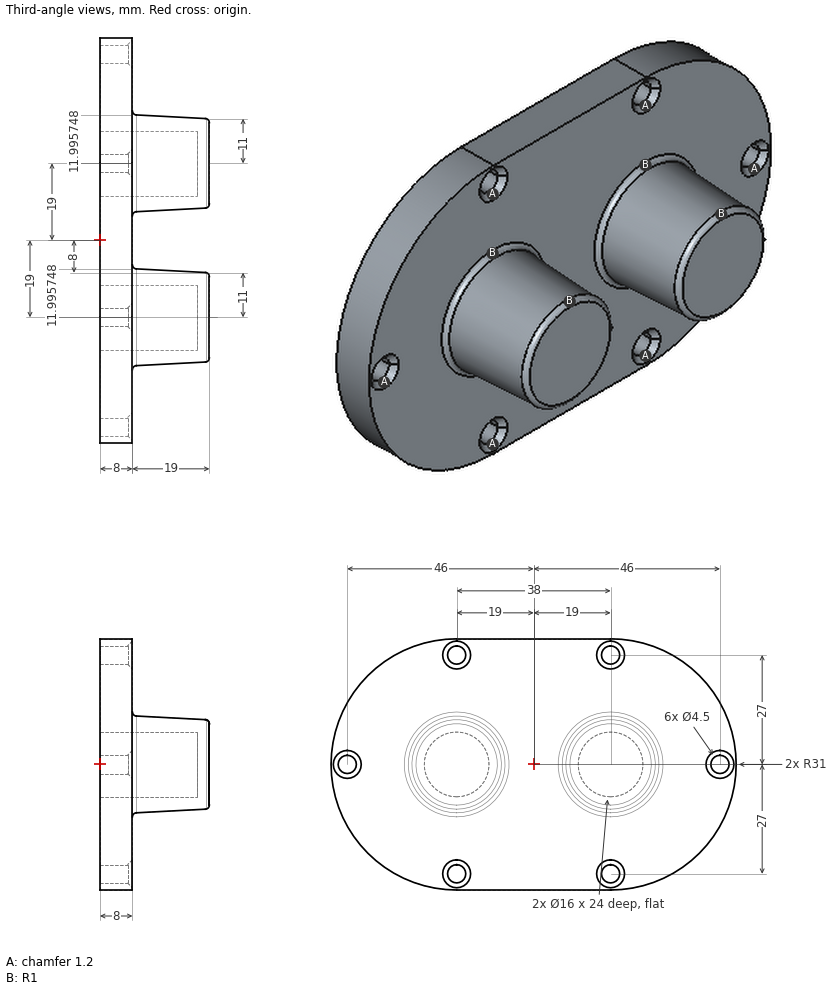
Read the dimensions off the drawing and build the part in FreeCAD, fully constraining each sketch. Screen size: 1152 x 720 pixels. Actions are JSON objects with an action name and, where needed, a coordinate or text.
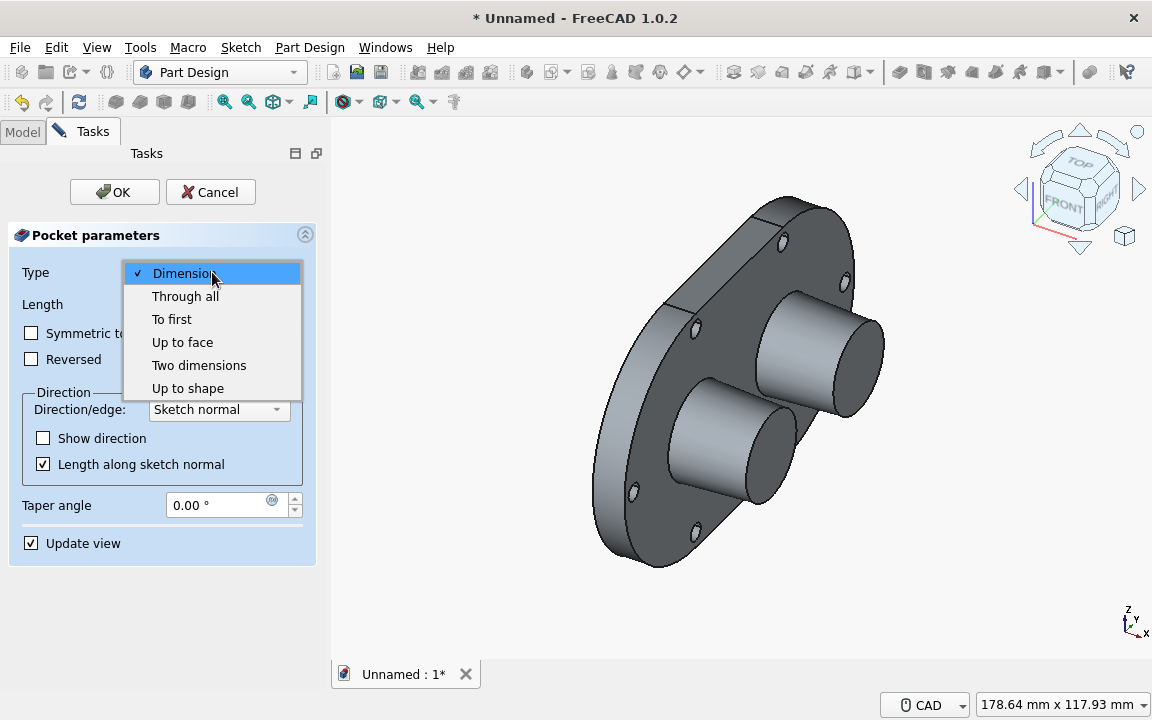
{"action": "left_click", "coordinate": [212, 296]}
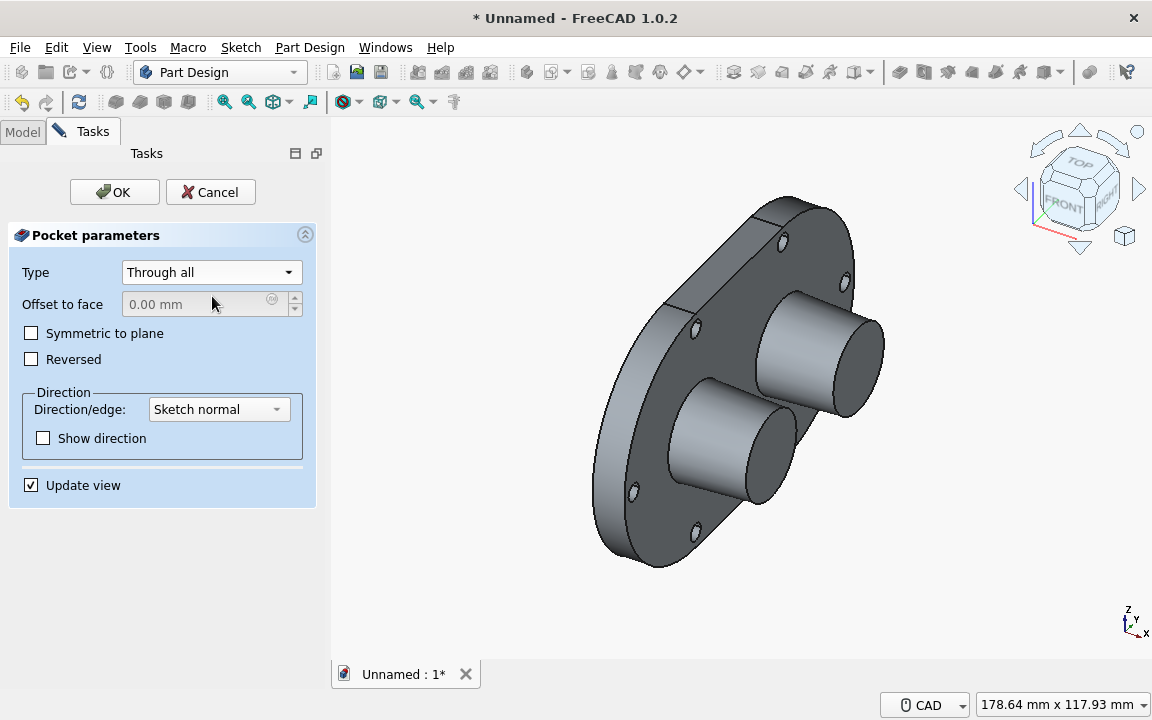
{"action": "left_click", "coordinate": [115, 192]}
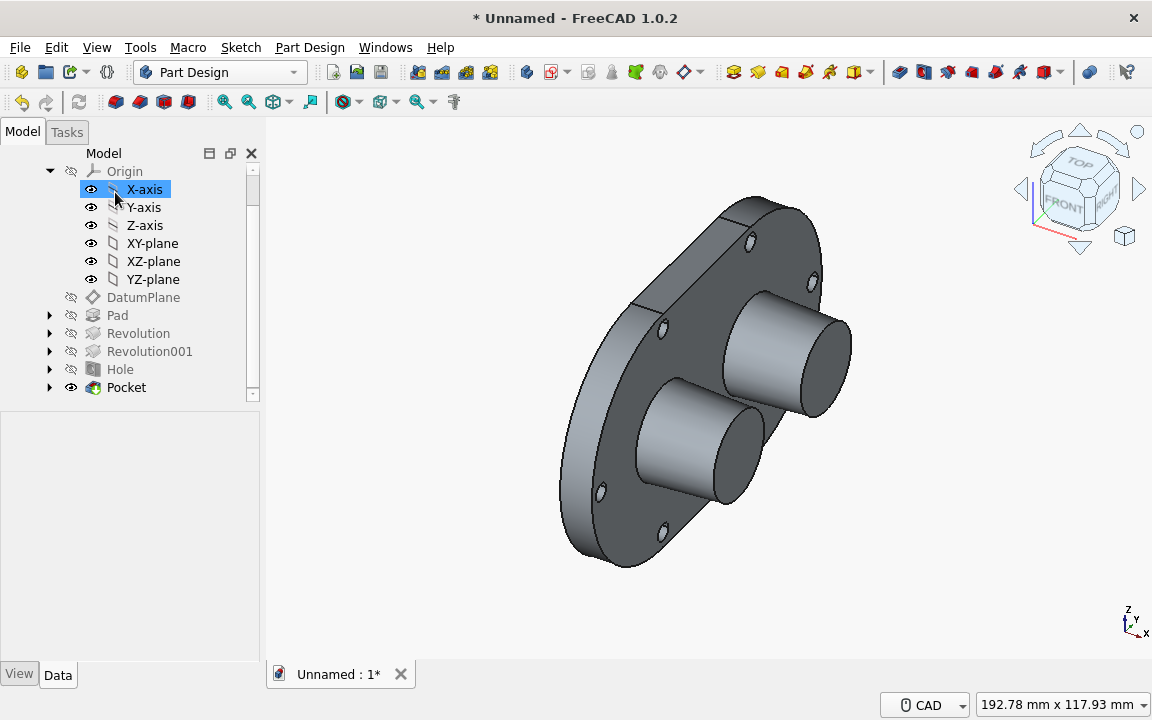
{"action": "left_click", "coordinate": [600, 501]}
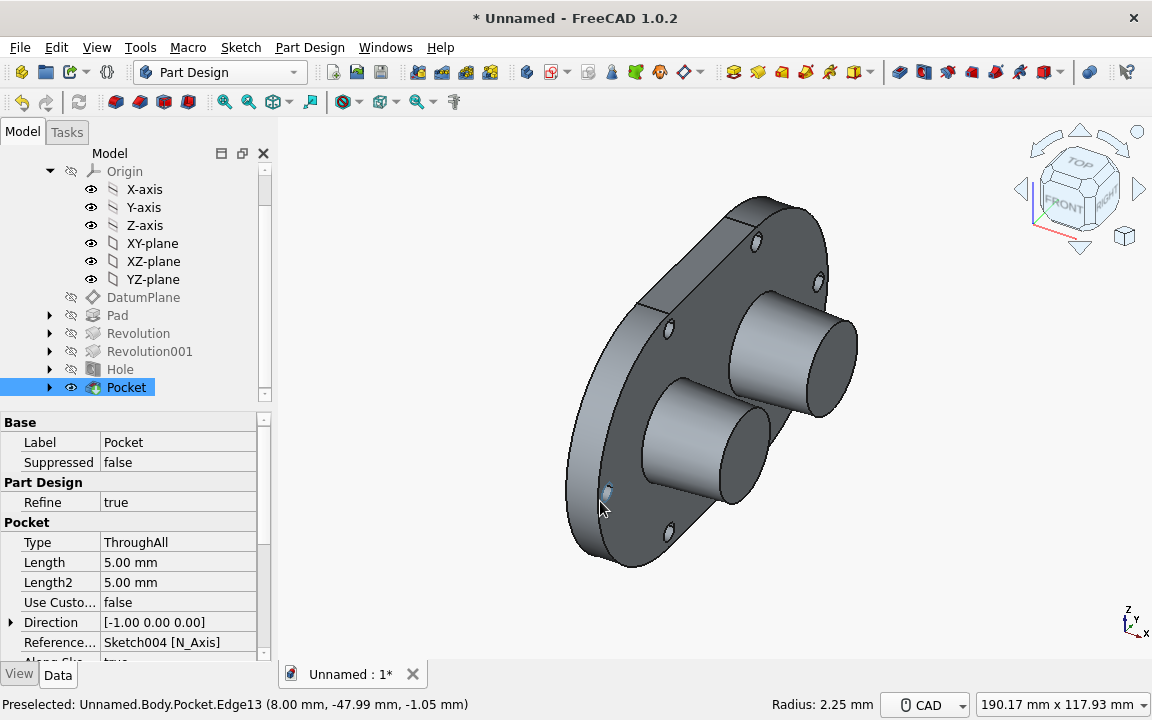
{"action": "left_click", "coordinate": [665, 540], "text": "ctrl"}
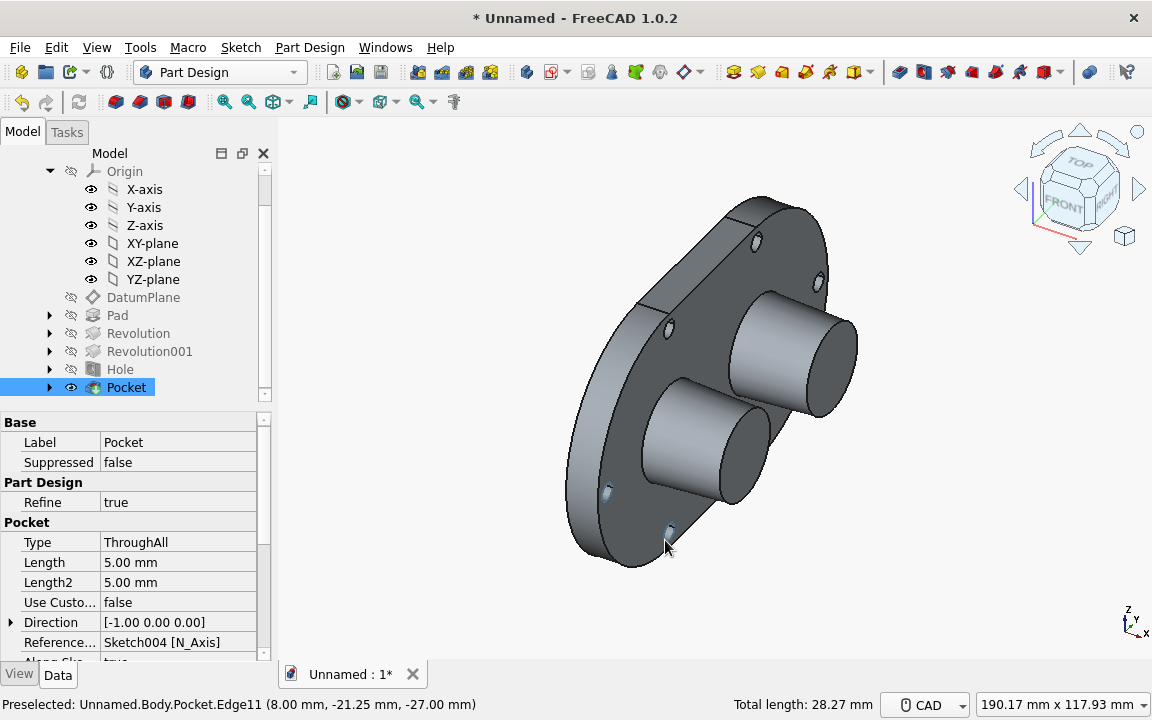
{"action": "left_click", "coordinate": [665, 337], "text": "ctrl"}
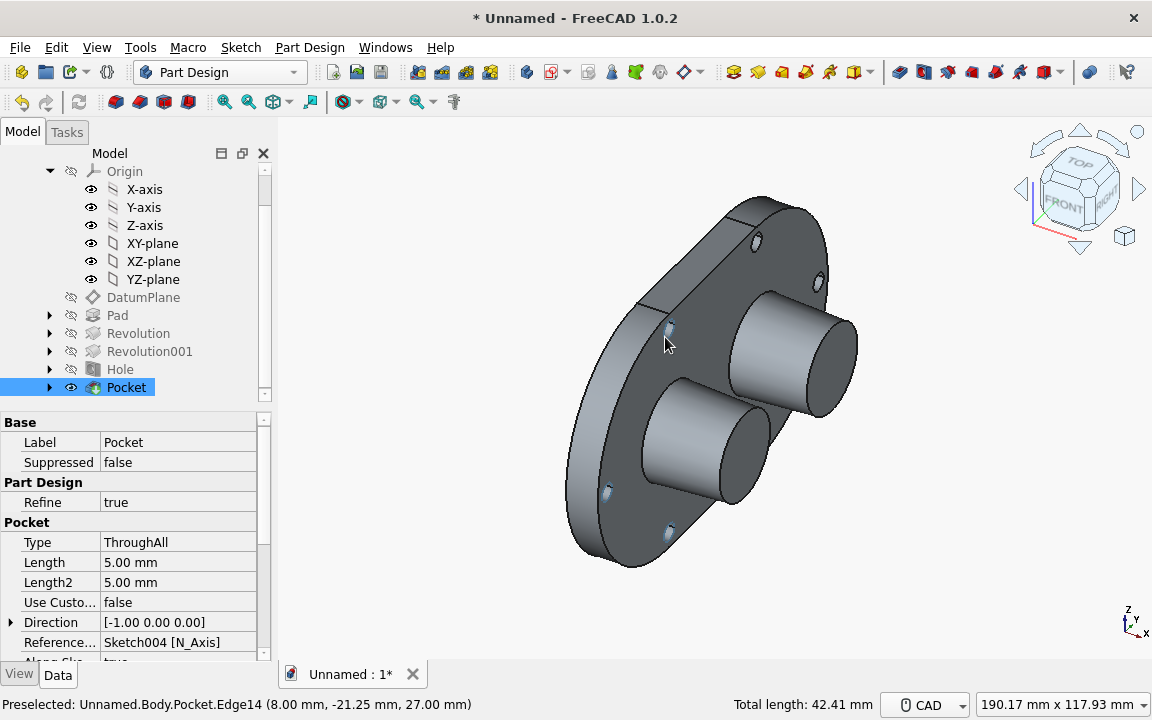
{"action": "left_click", "coordinate": [752, 250], "text": "ctrl"}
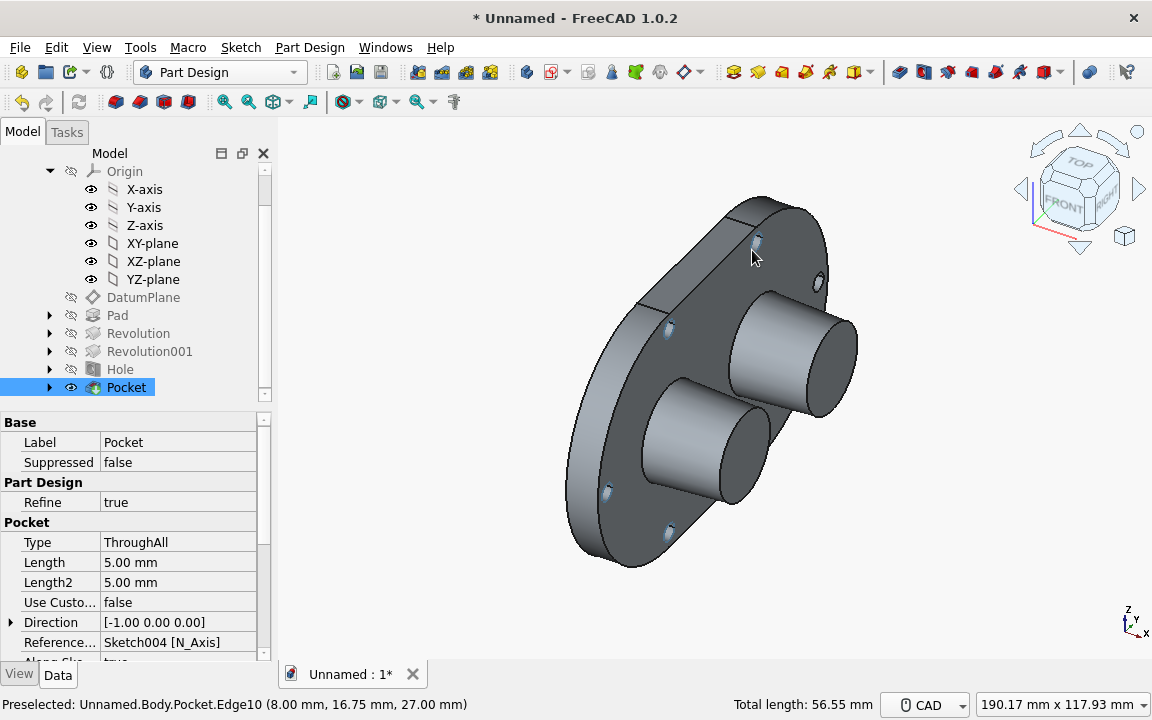
{"action": "left_click", "coordinate": [814, 290], "text": "ctrl"}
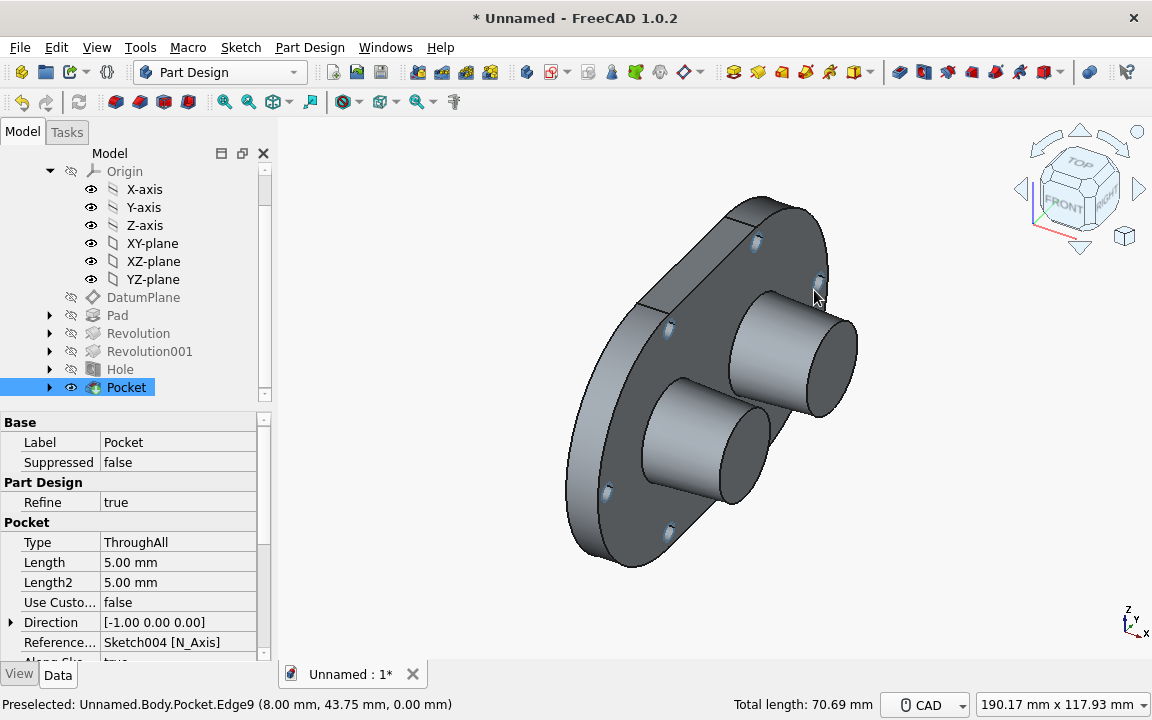
{"action": "key", "text": "0"}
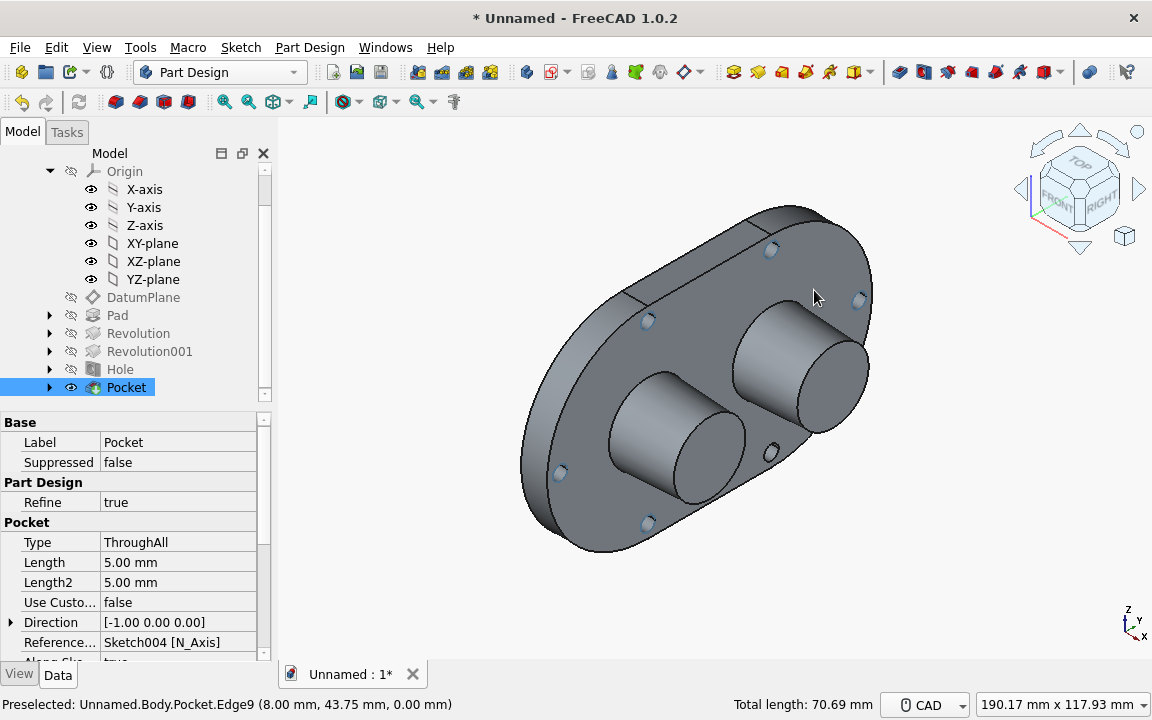
{"action": "left_click", "coordinate": [764, 456], "text": "ctrl"}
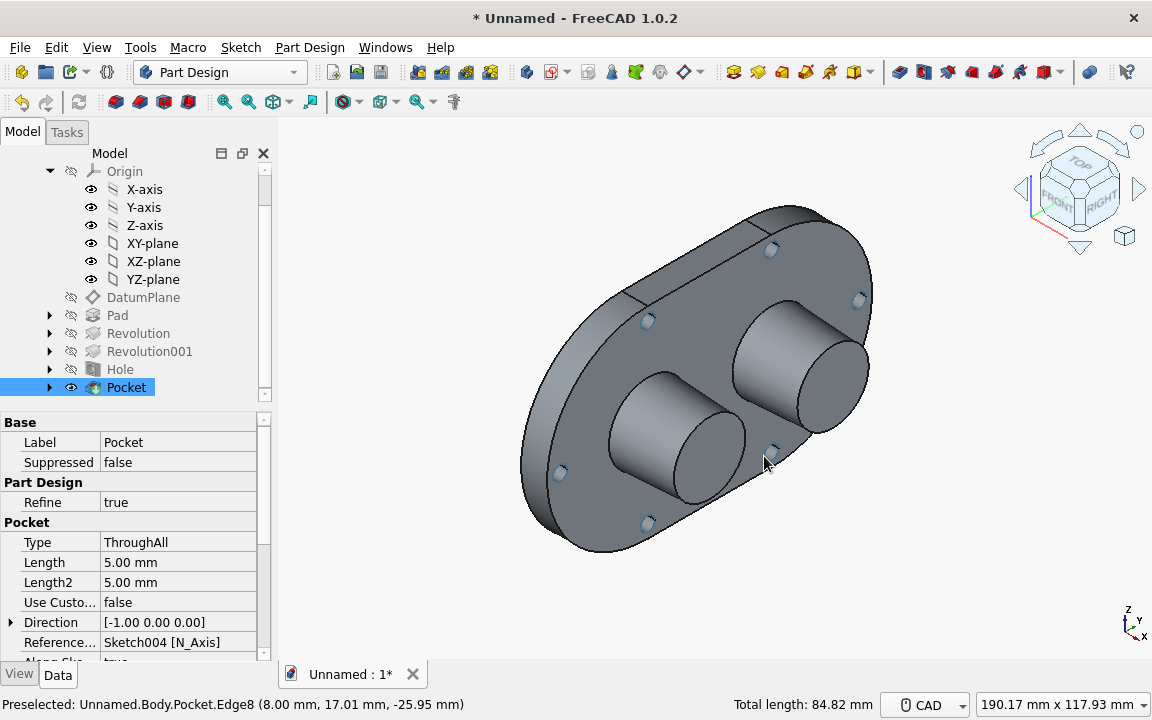
{"action": "left_click", "coordinate": [140, 102]}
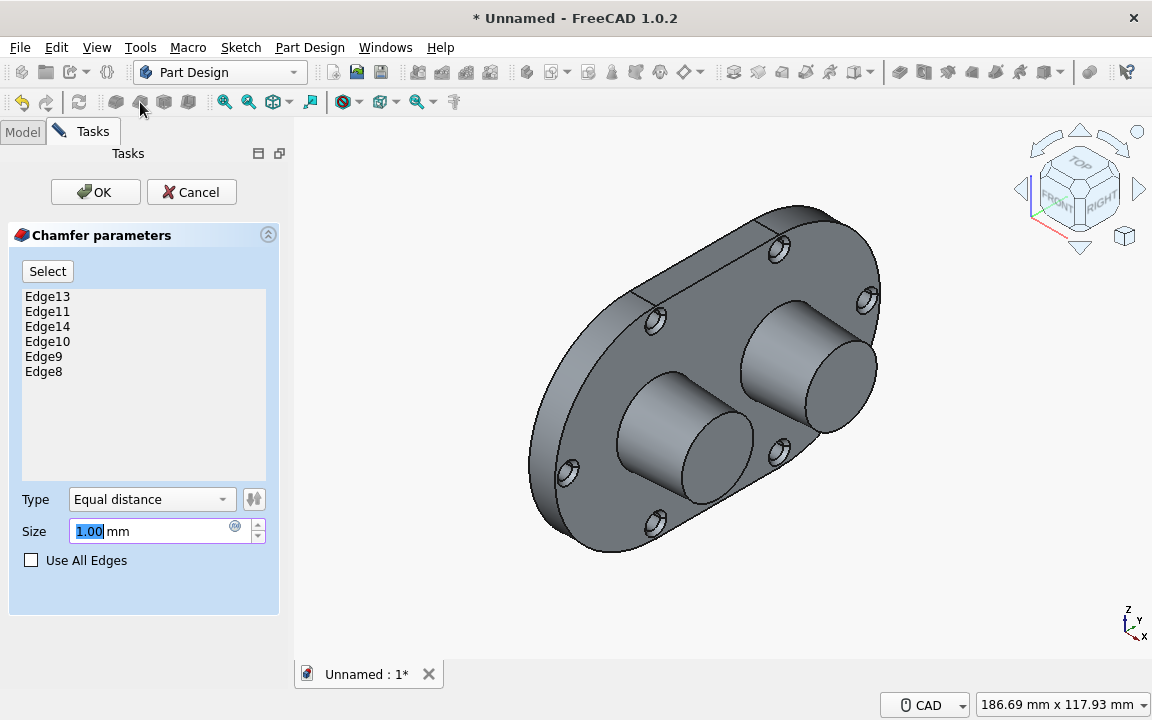
{"action": "type", "text": "1.2"}
{"action": "key", "text": "Tab"}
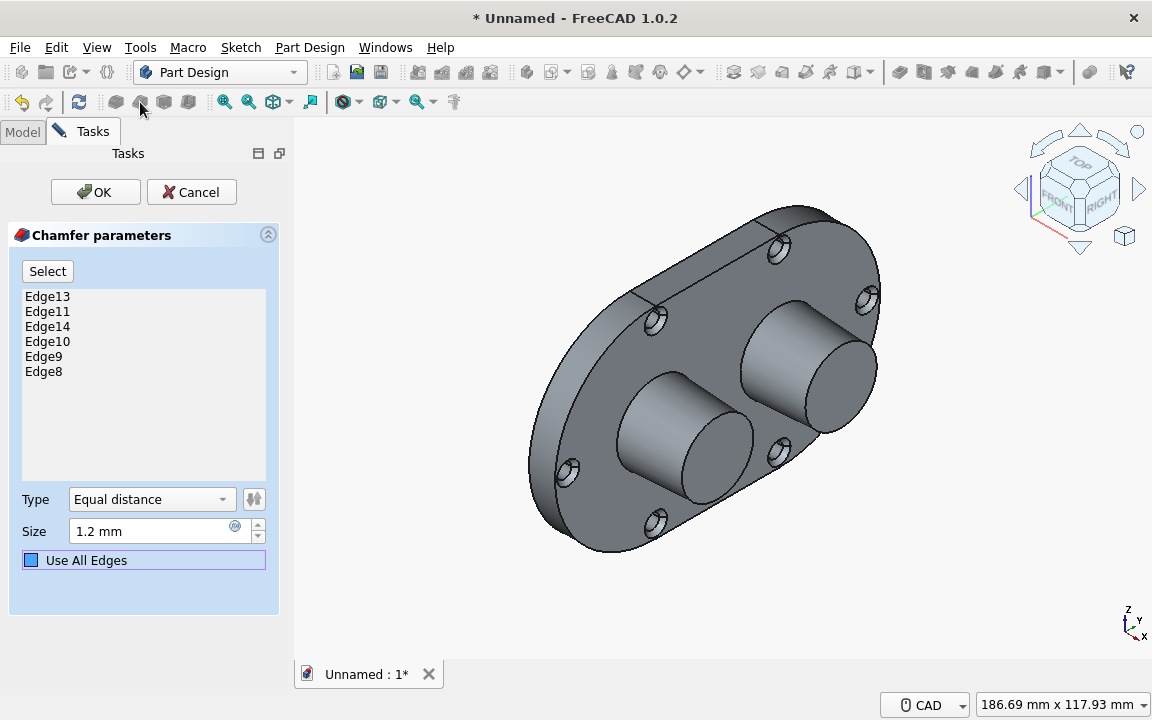
{"action": "left_click", "coordinate": [96, 192]}